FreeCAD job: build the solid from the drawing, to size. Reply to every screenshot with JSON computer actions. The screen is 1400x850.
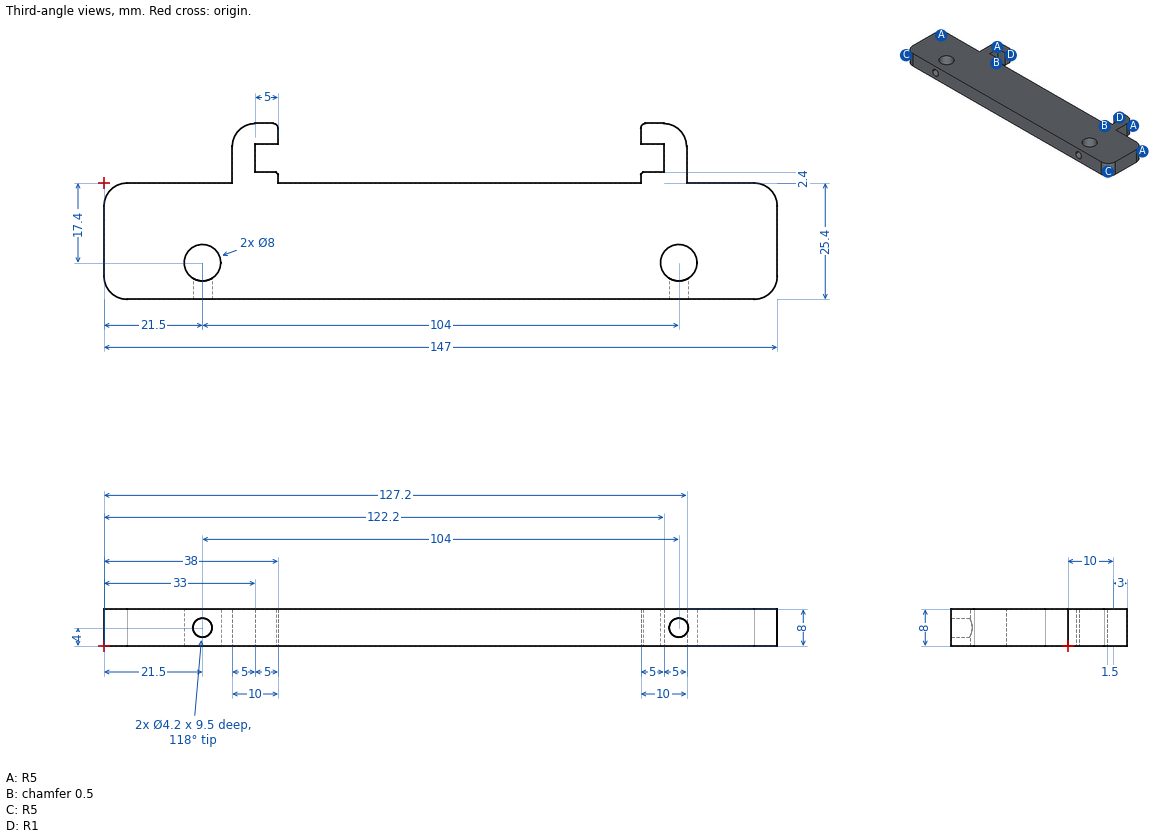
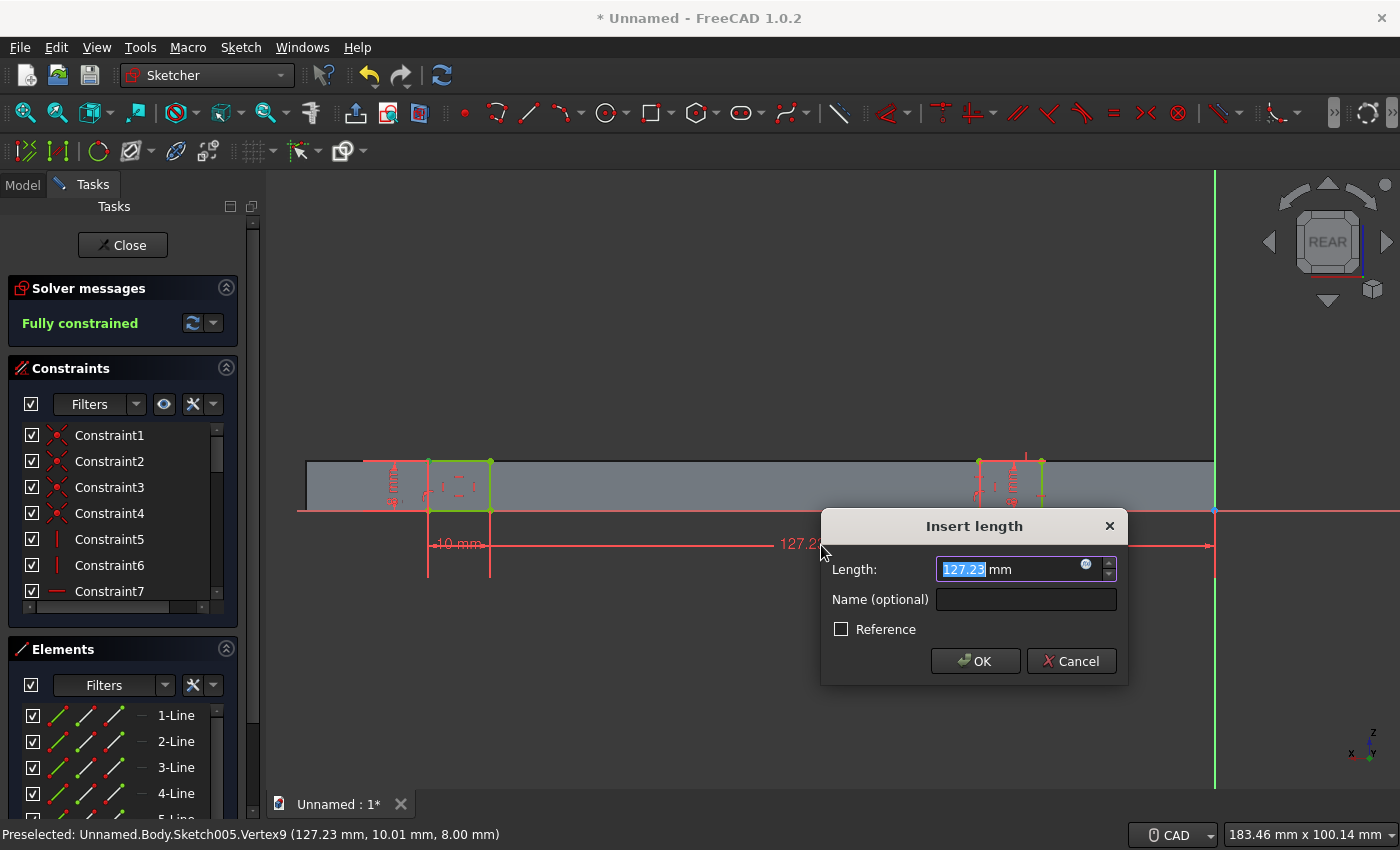
{"action": "type", "text": "127.2"}
{"action": "key", "text": "Return"}
{"action": "key", "text": "Escape"}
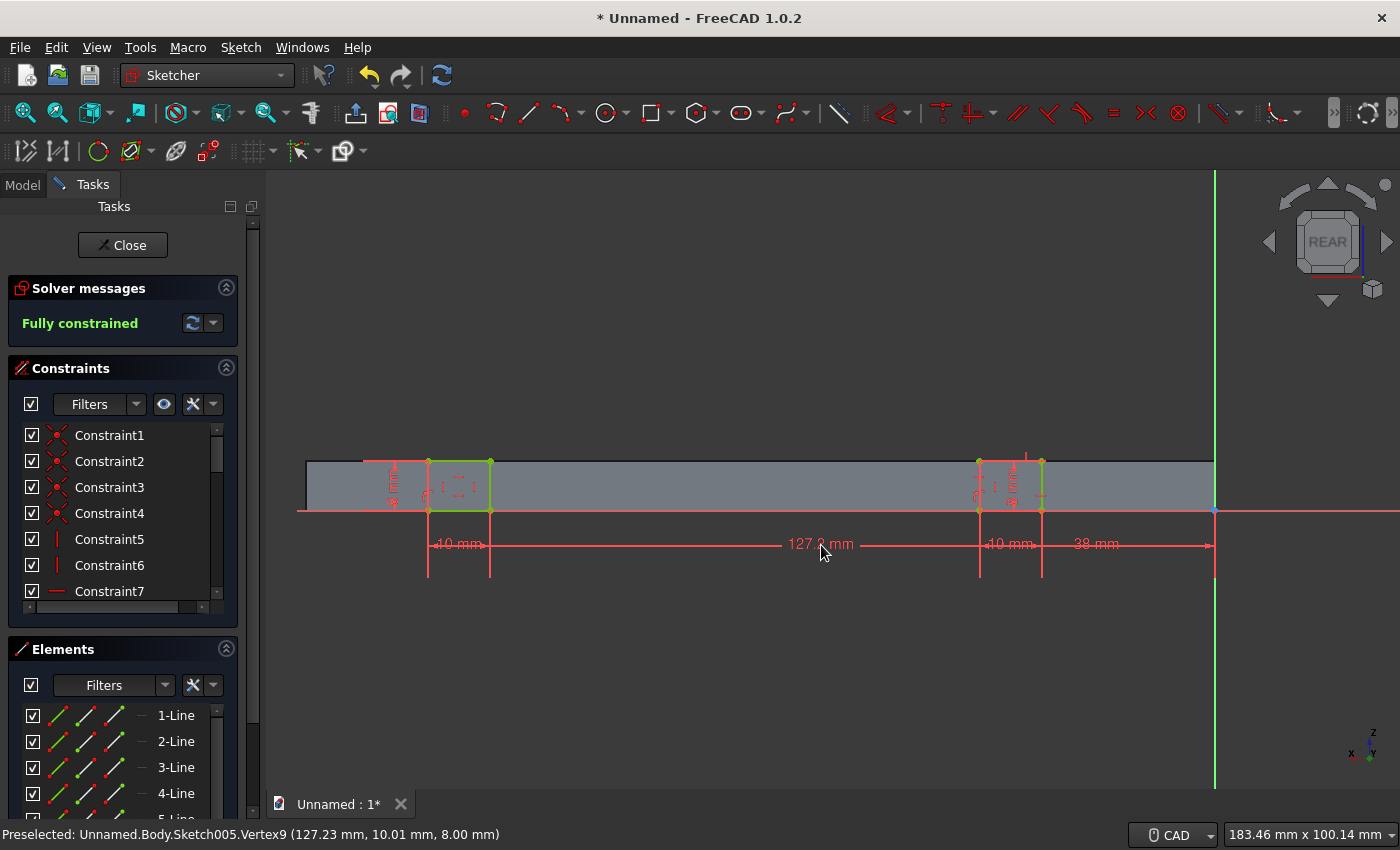
{"action": "left_click", "coordinate": [123, 245]}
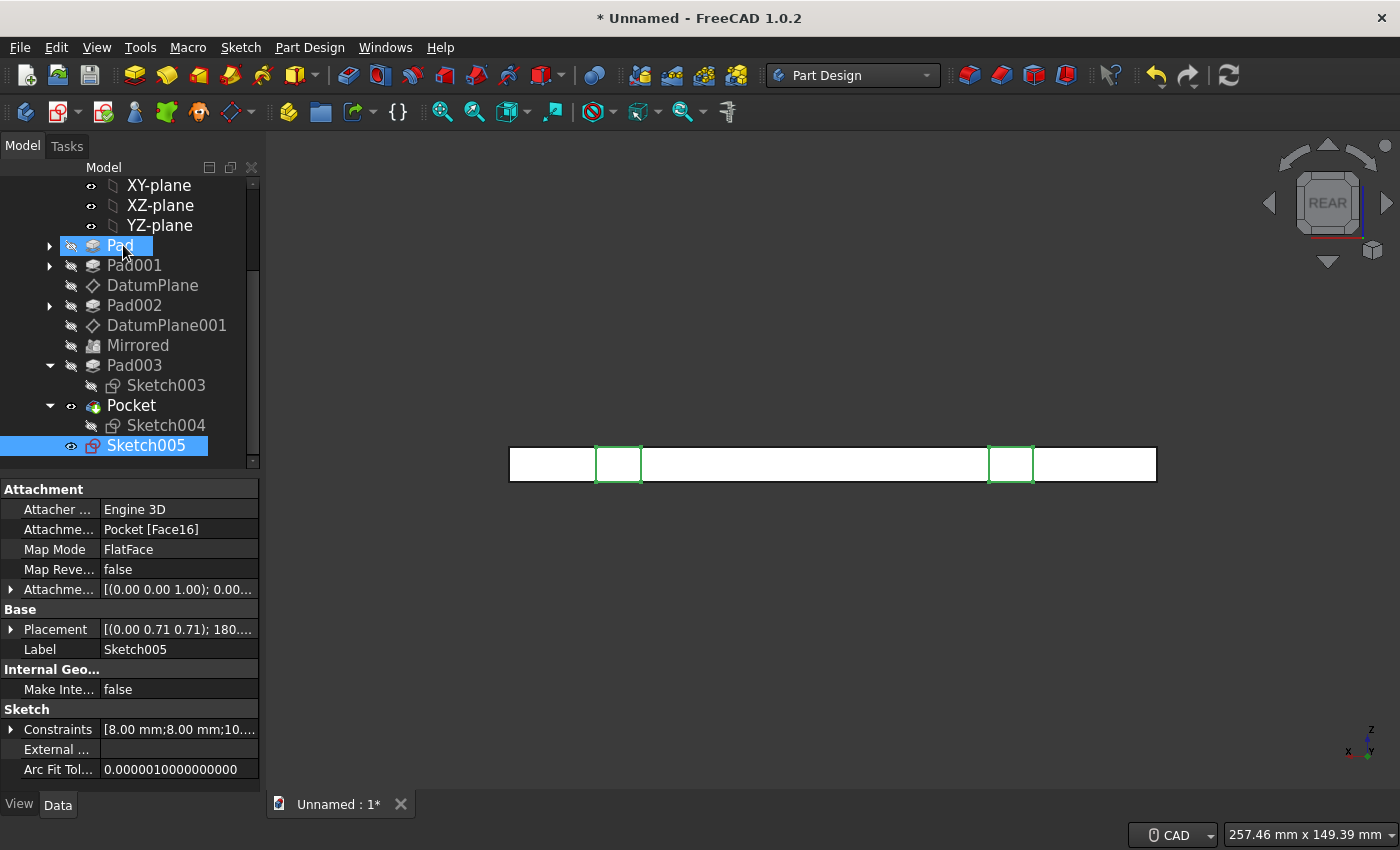
{"action": "left_click", "coordinate": [136, 76]}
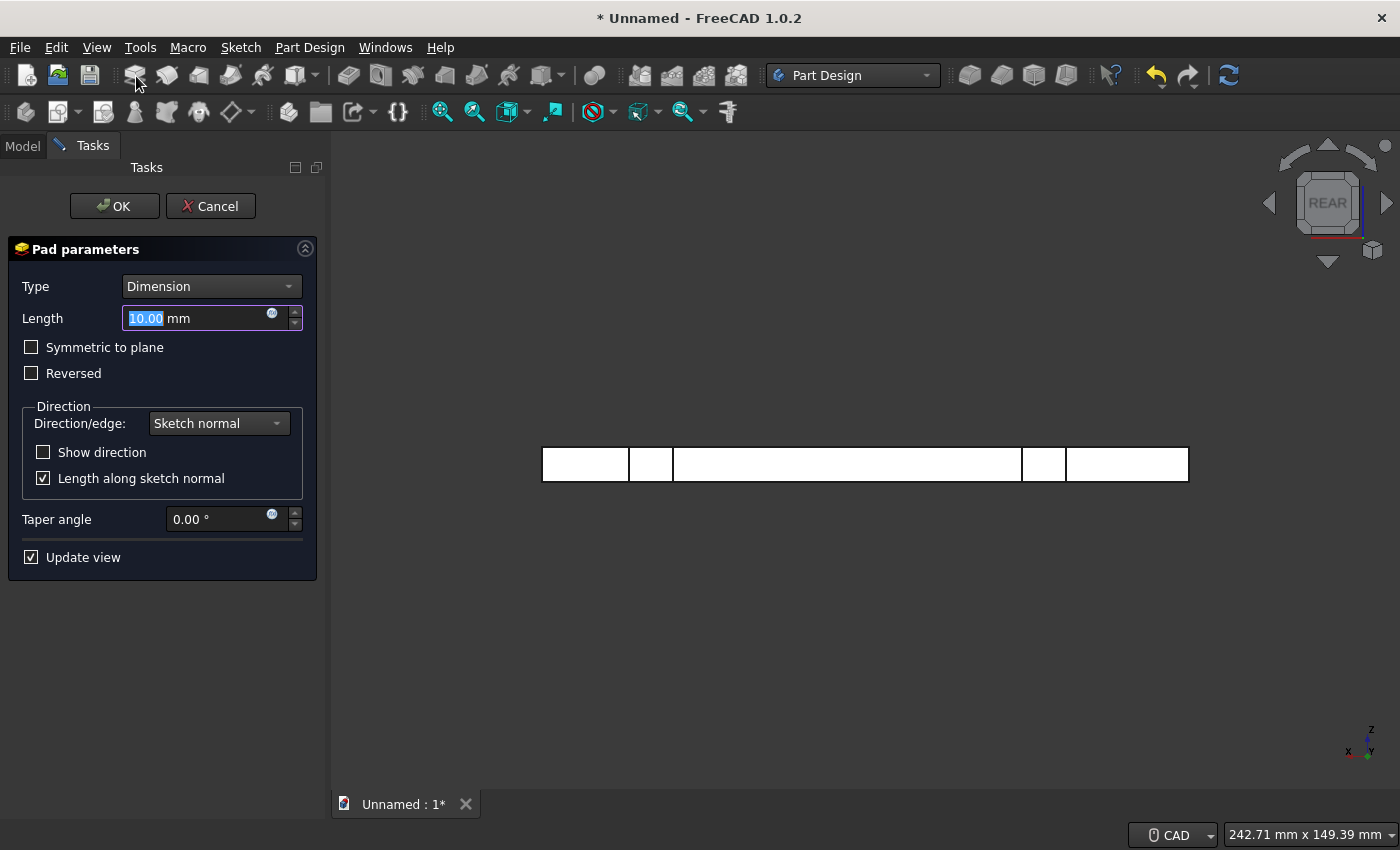
{"action": "type", "text": "3"}
{"action": "key", "text": "Tab"}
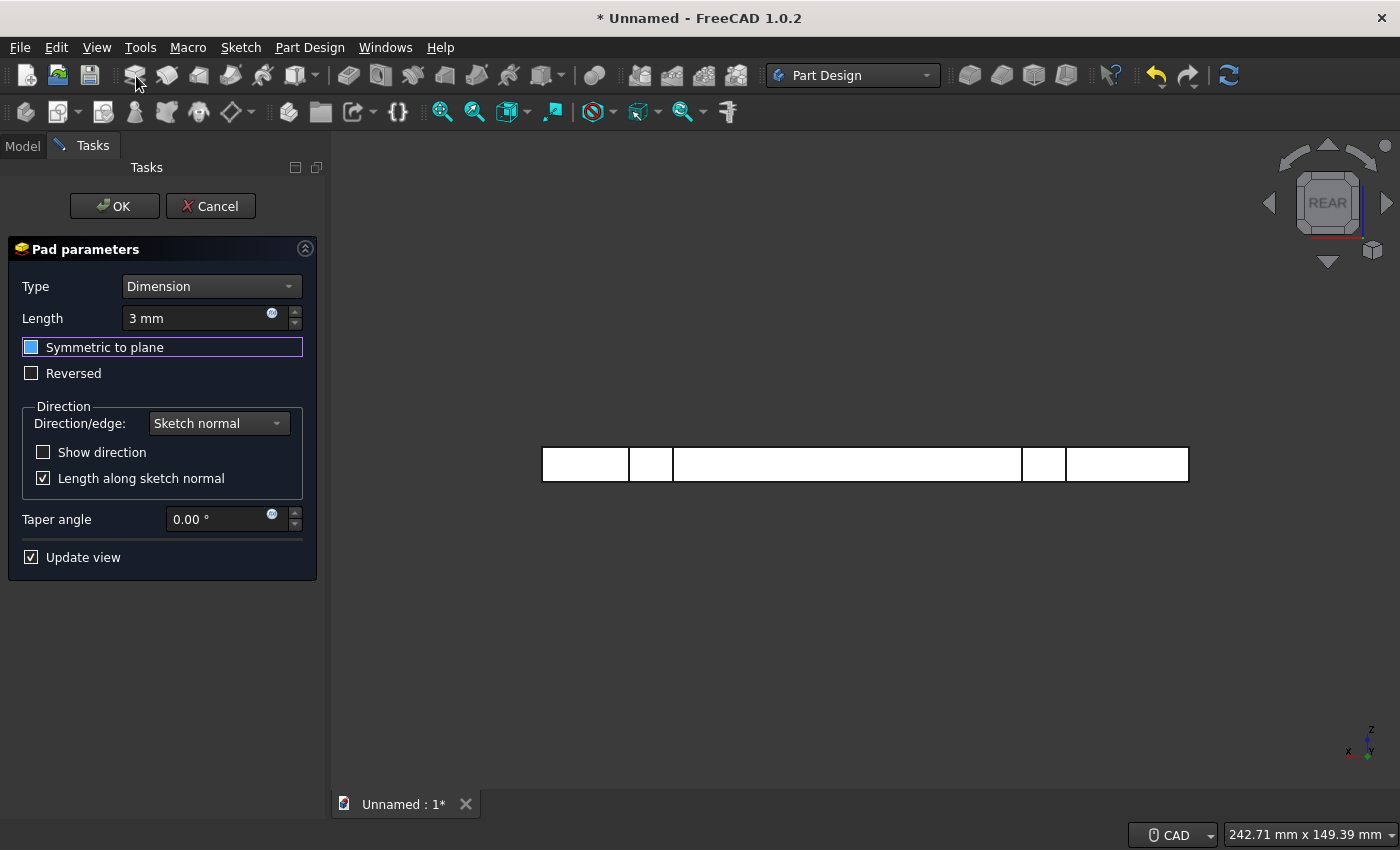
{"action": "left_click", "coordinate": [115, 206]}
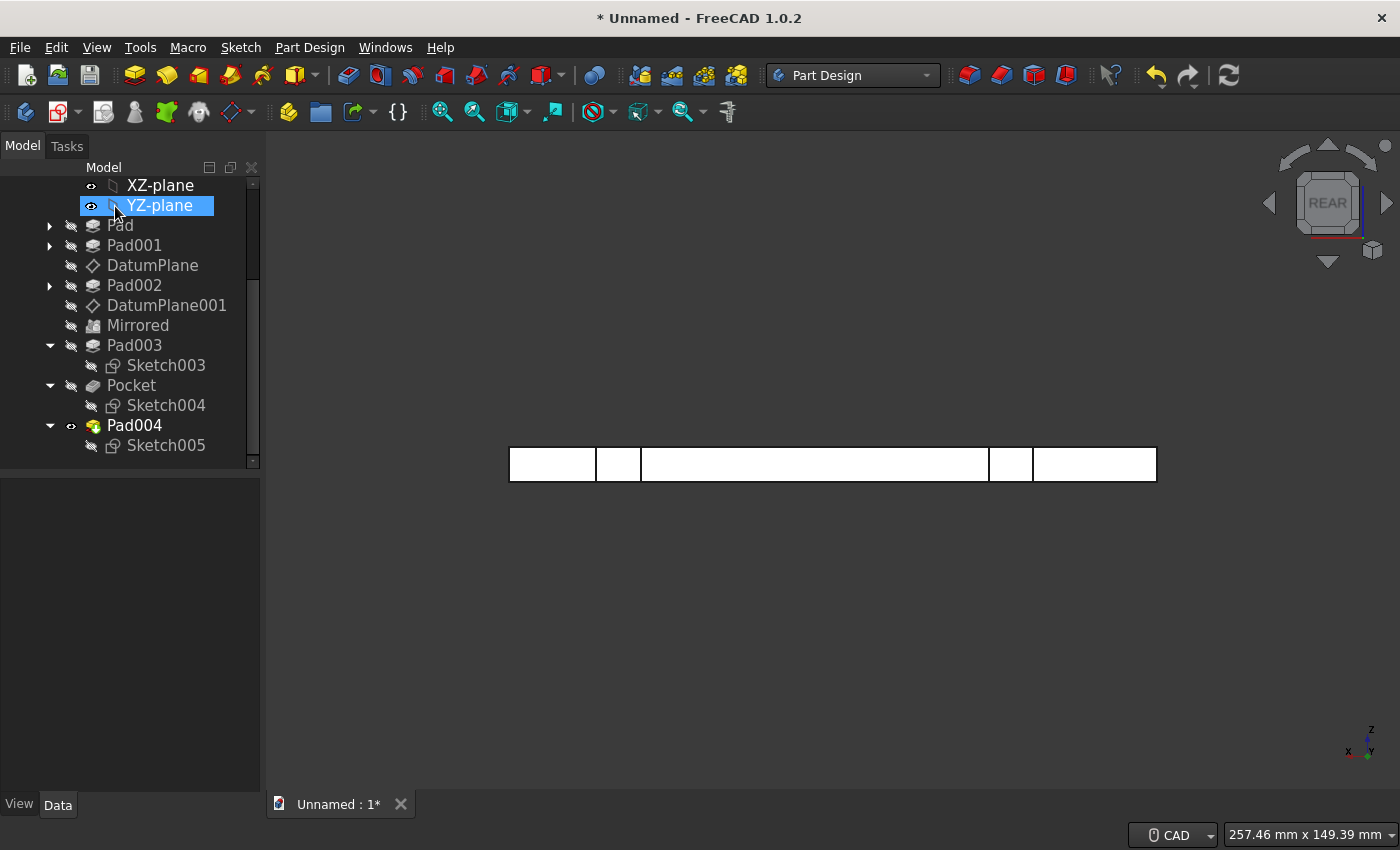
{"action": "left_click", "coordinate": [1033, 463]}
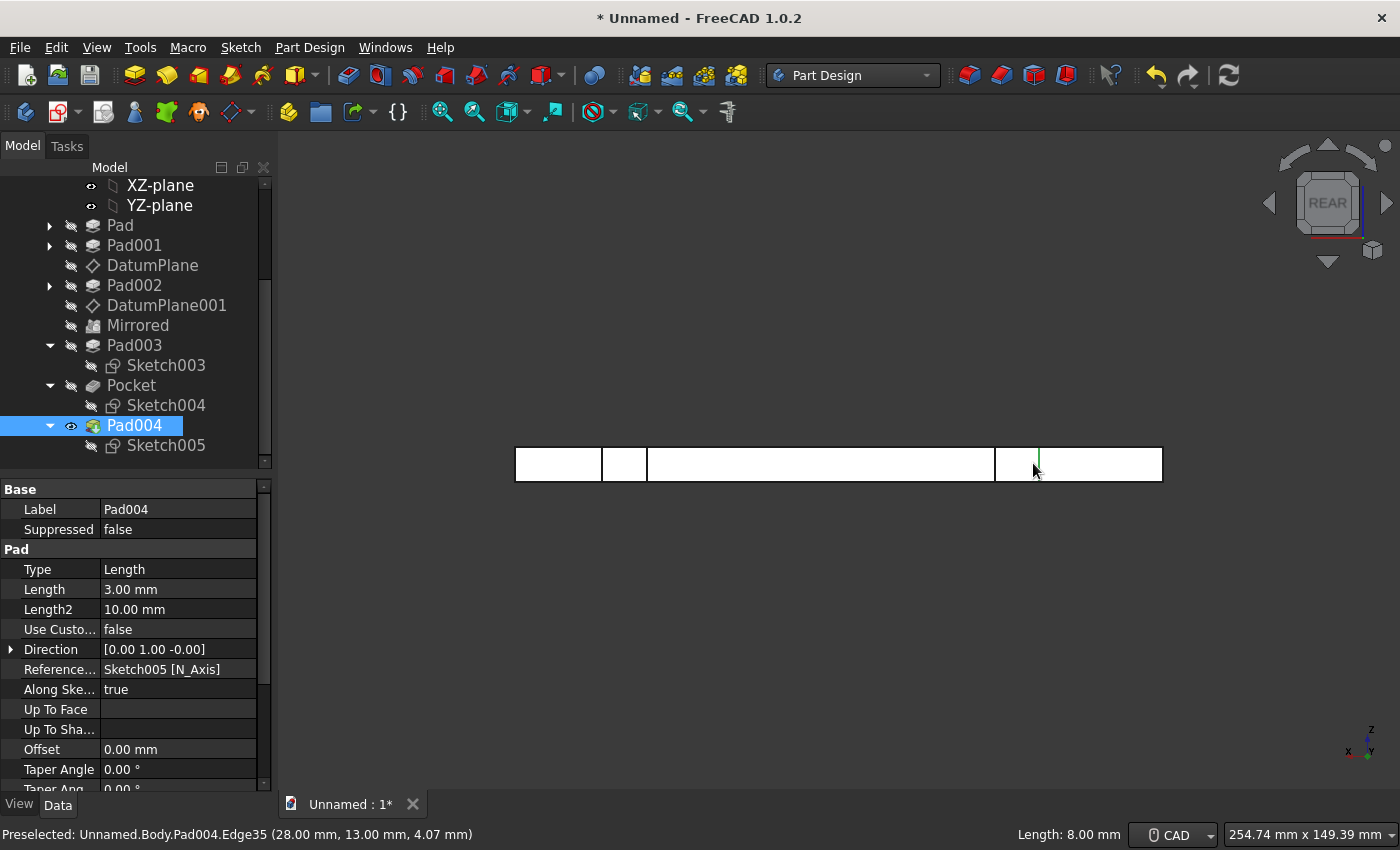
{"action": "left_click", "coordinate": [1163, 463], "text": "ctrl"}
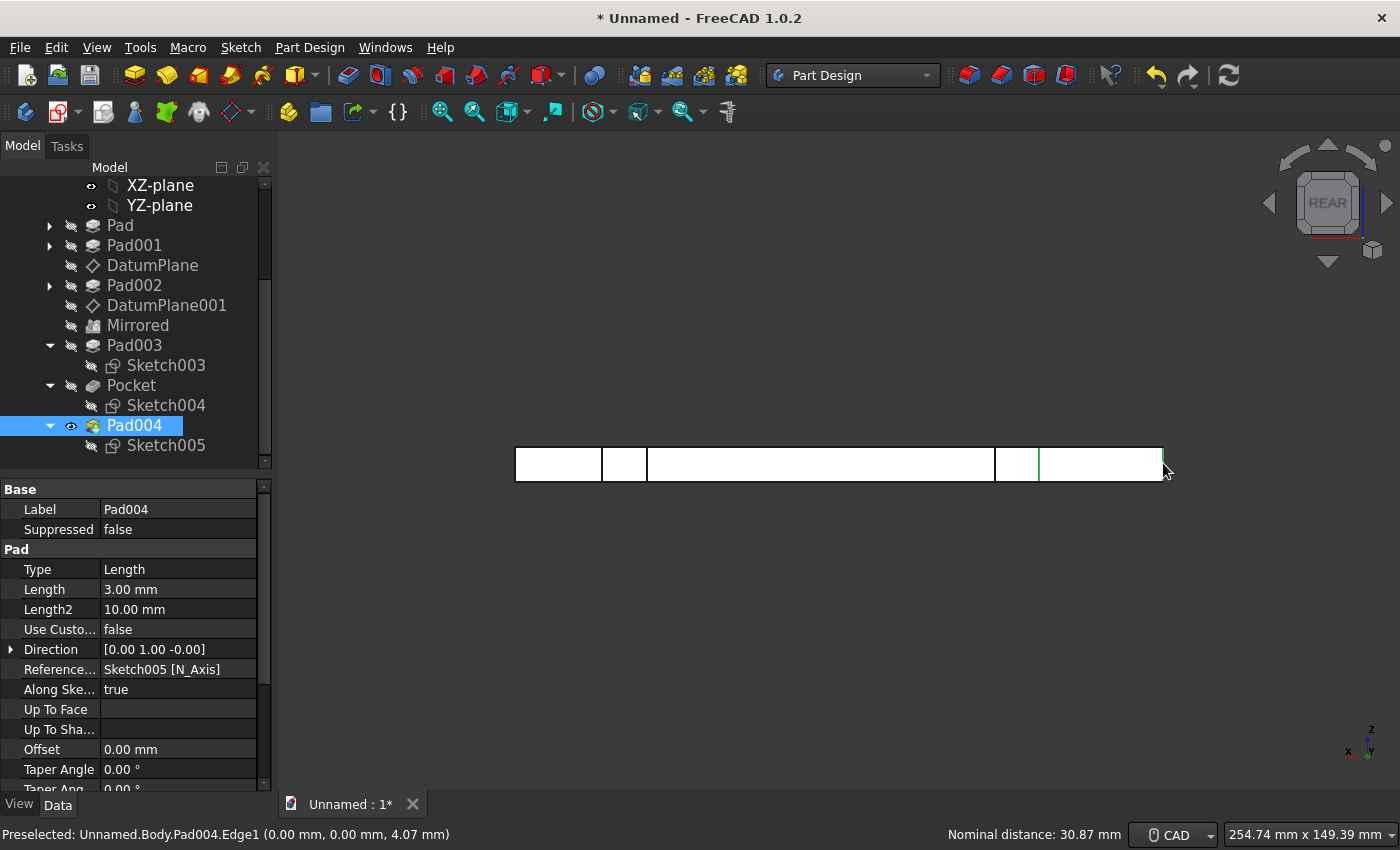
{"action": "key", "text": "0"}